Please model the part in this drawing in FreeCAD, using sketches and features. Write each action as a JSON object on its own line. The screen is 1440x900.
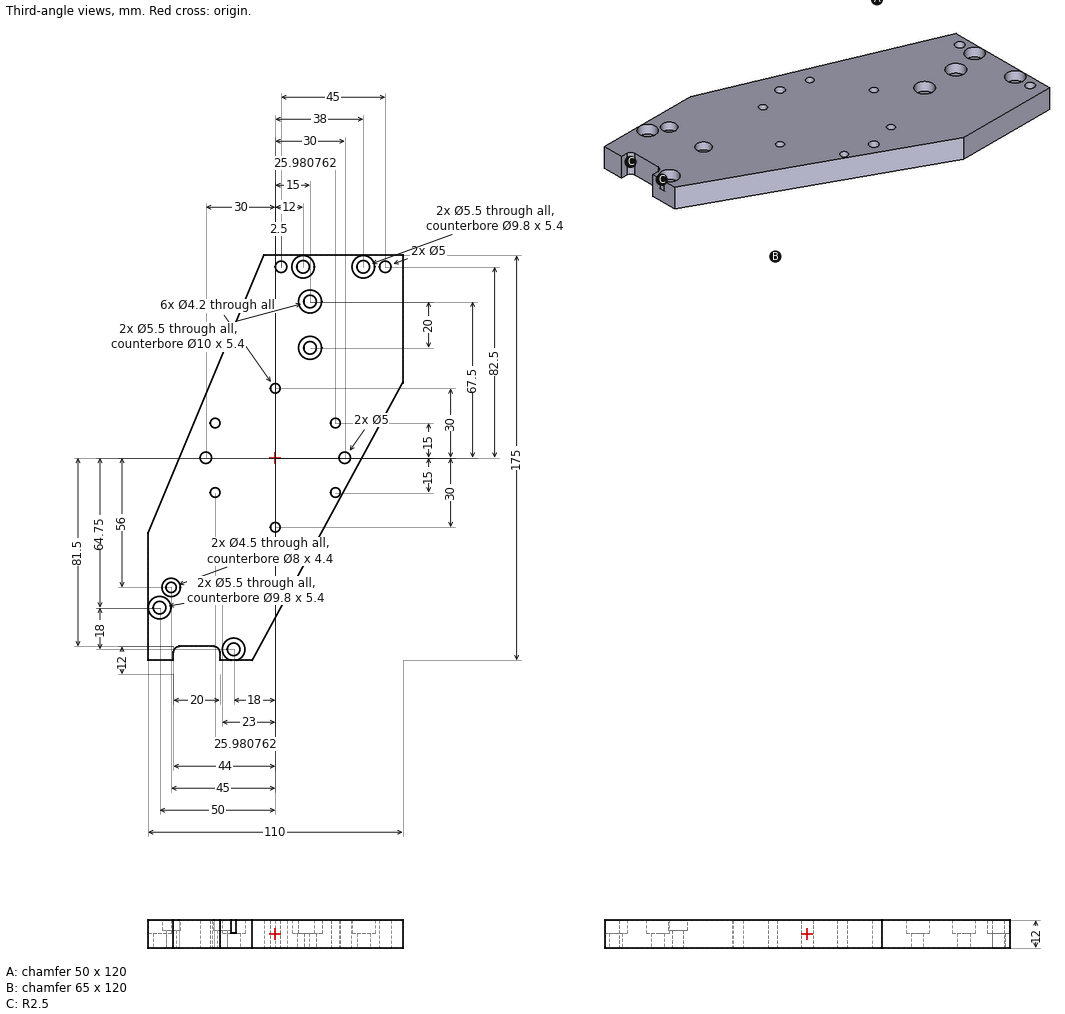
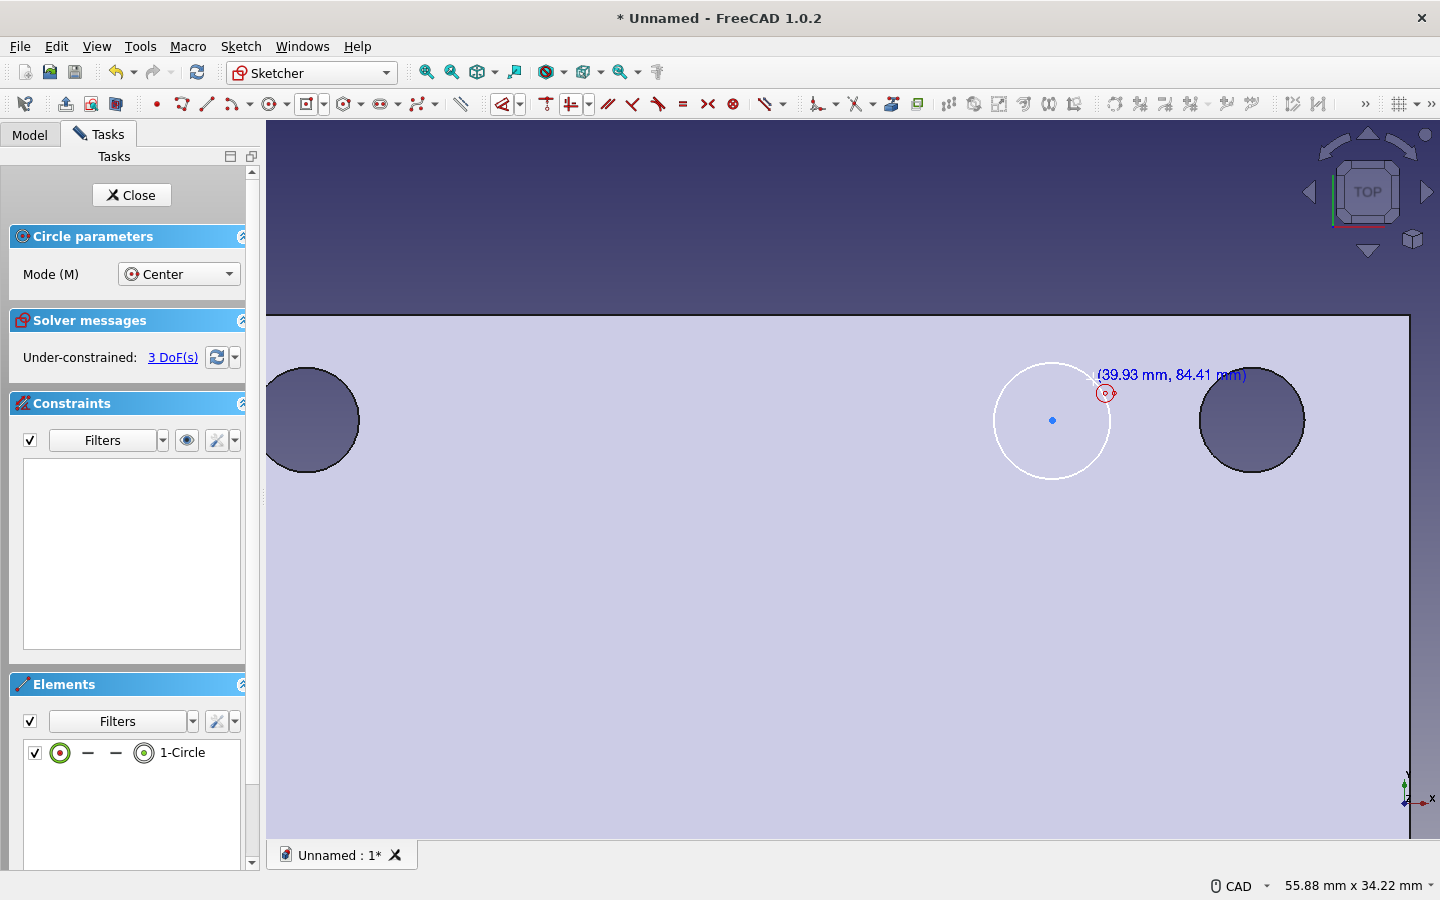
{"action": "left_click", "coordinate": [506, 420]}
{"action": "left_click", "coordinate": [547, 379]}
{"action": "key", "text": "Escape"}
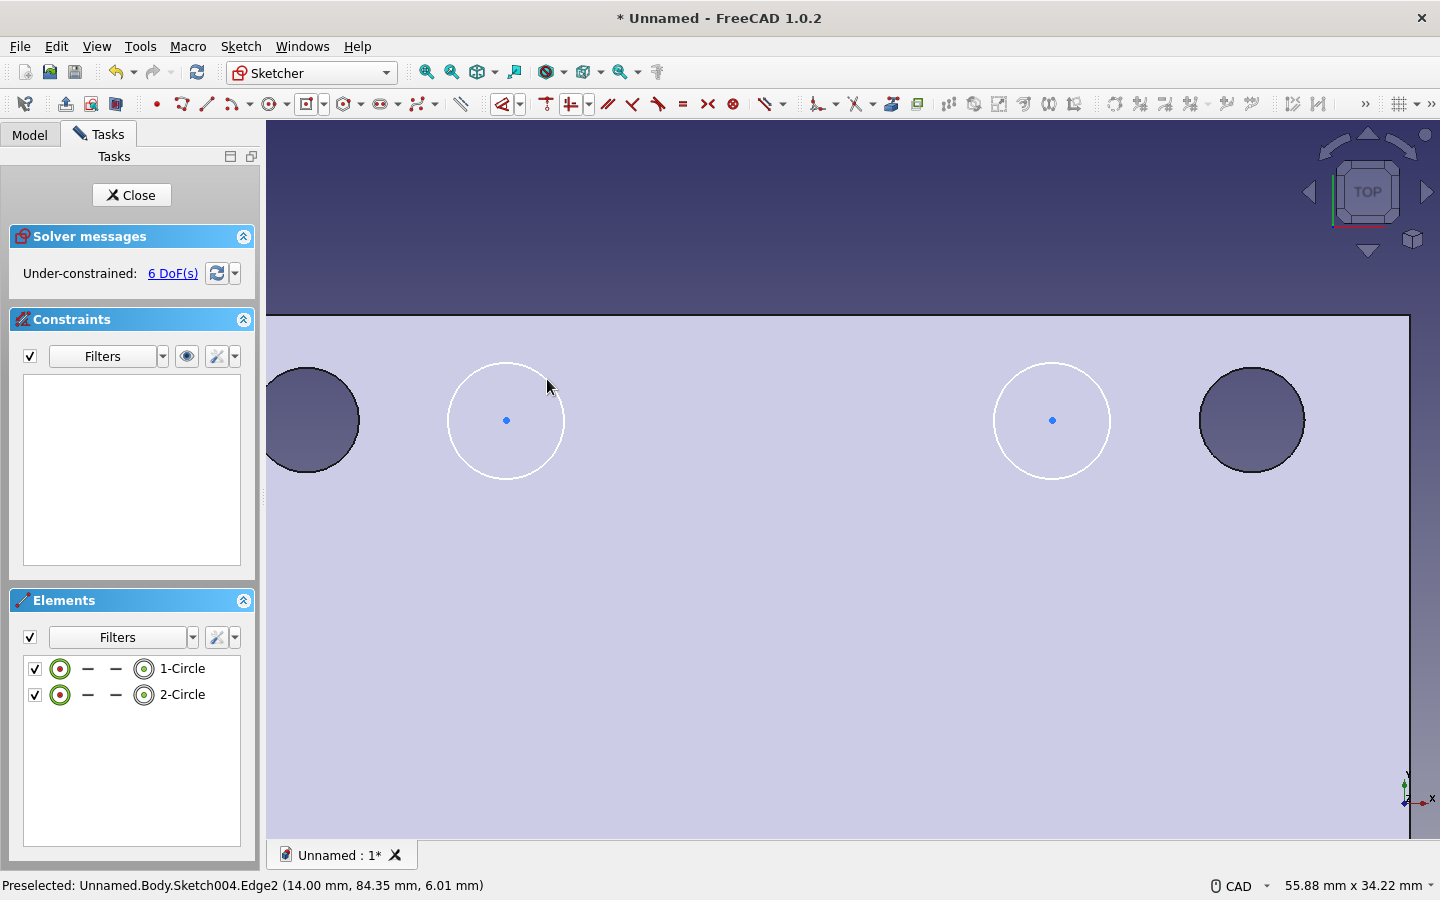
{"action": "left_click", "coordinate": [1093, 380]}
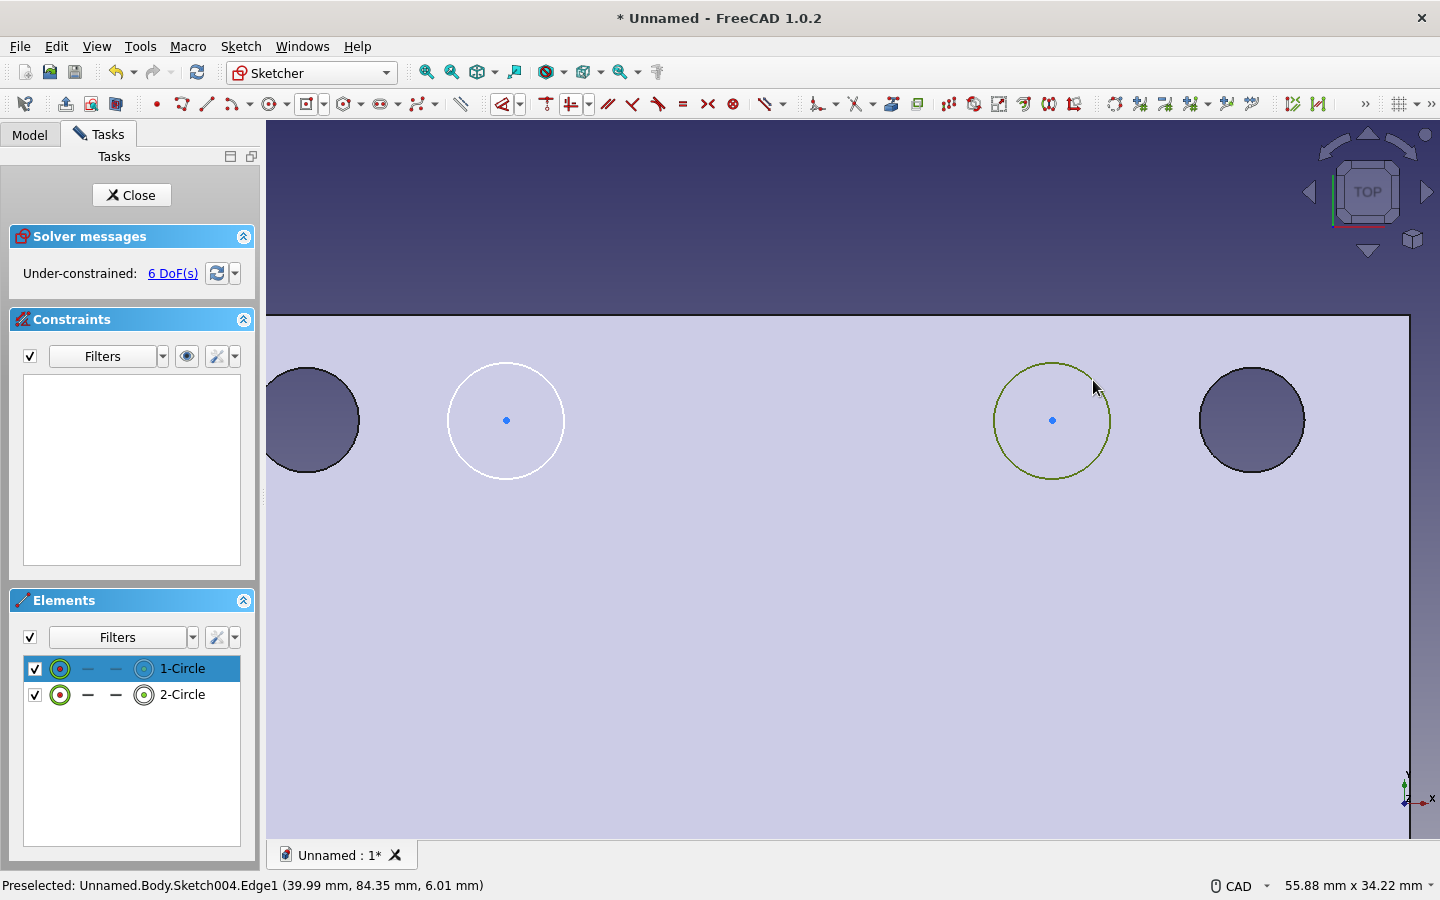
{"action": "left_click", "coordinate": [547, 380]}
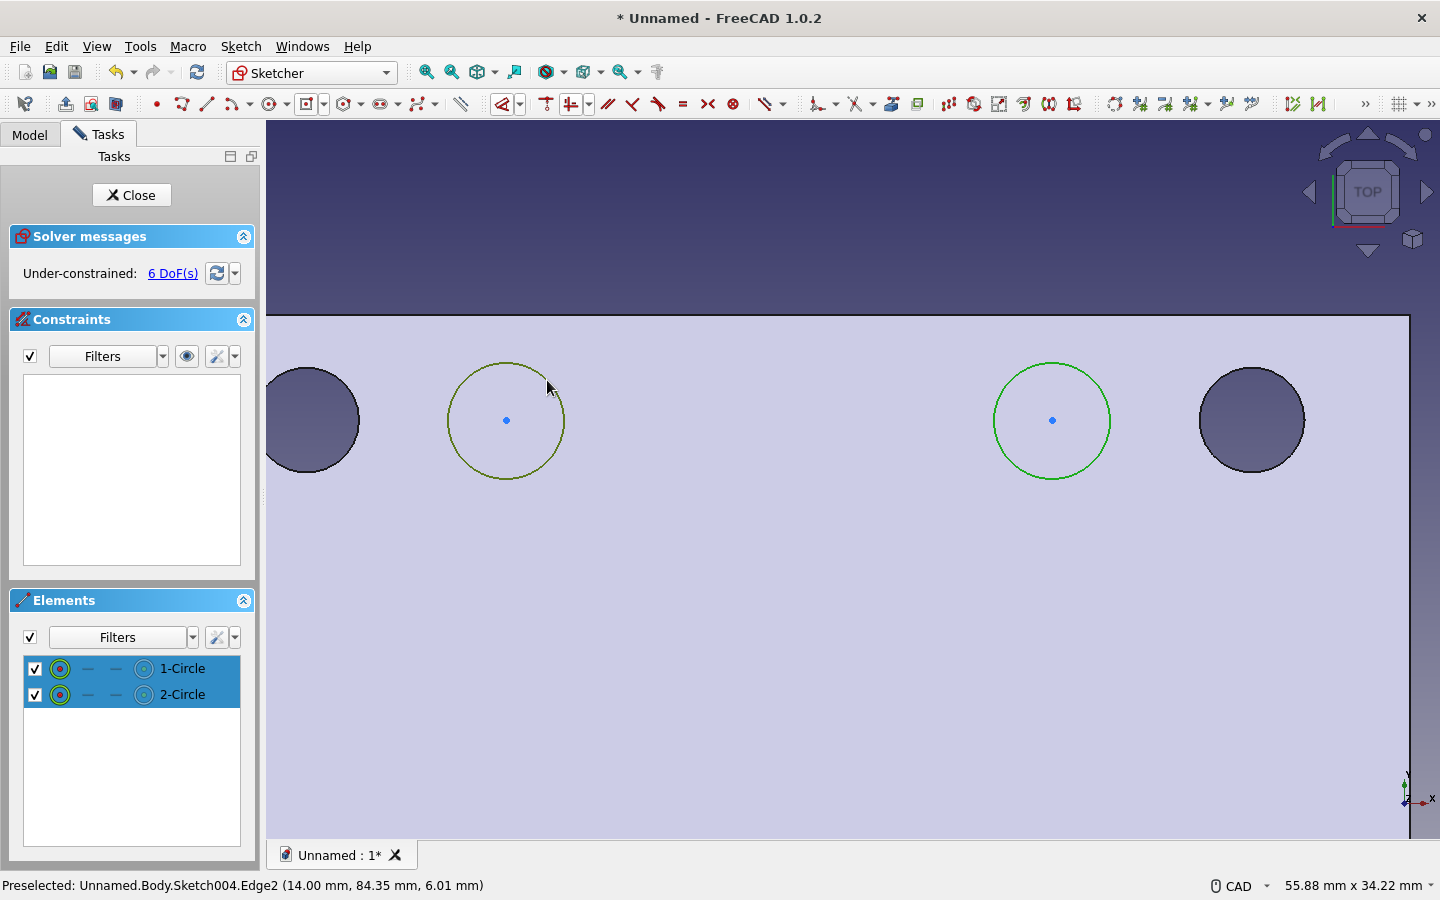
{"action": "key", "text": "e"}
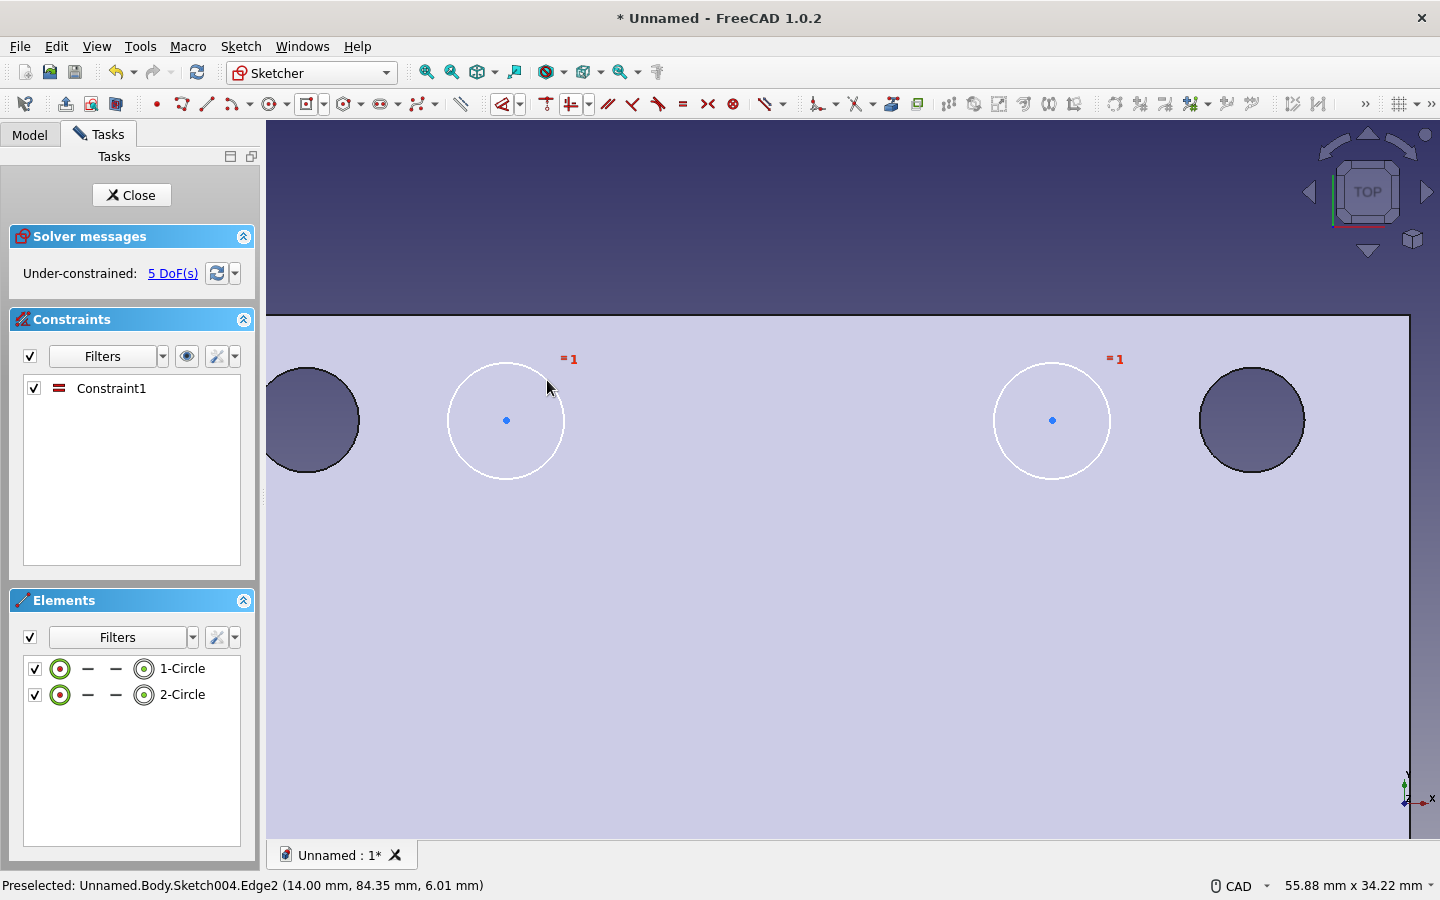
{"action": "left_click", "coordinate": [1052, 421]}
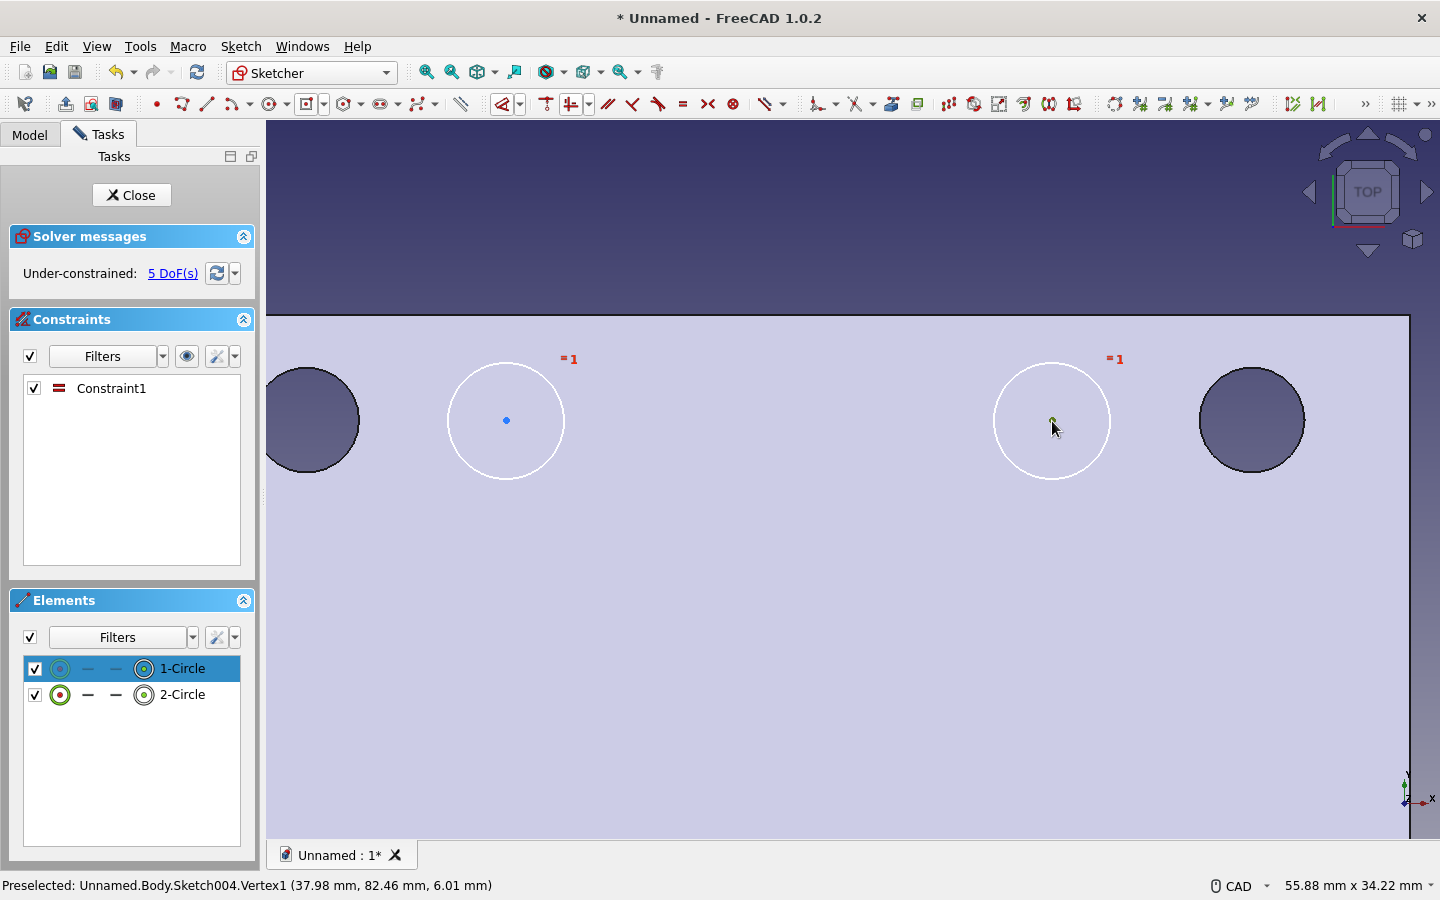
{"action": "left_click", "coordinate": [506, 421]}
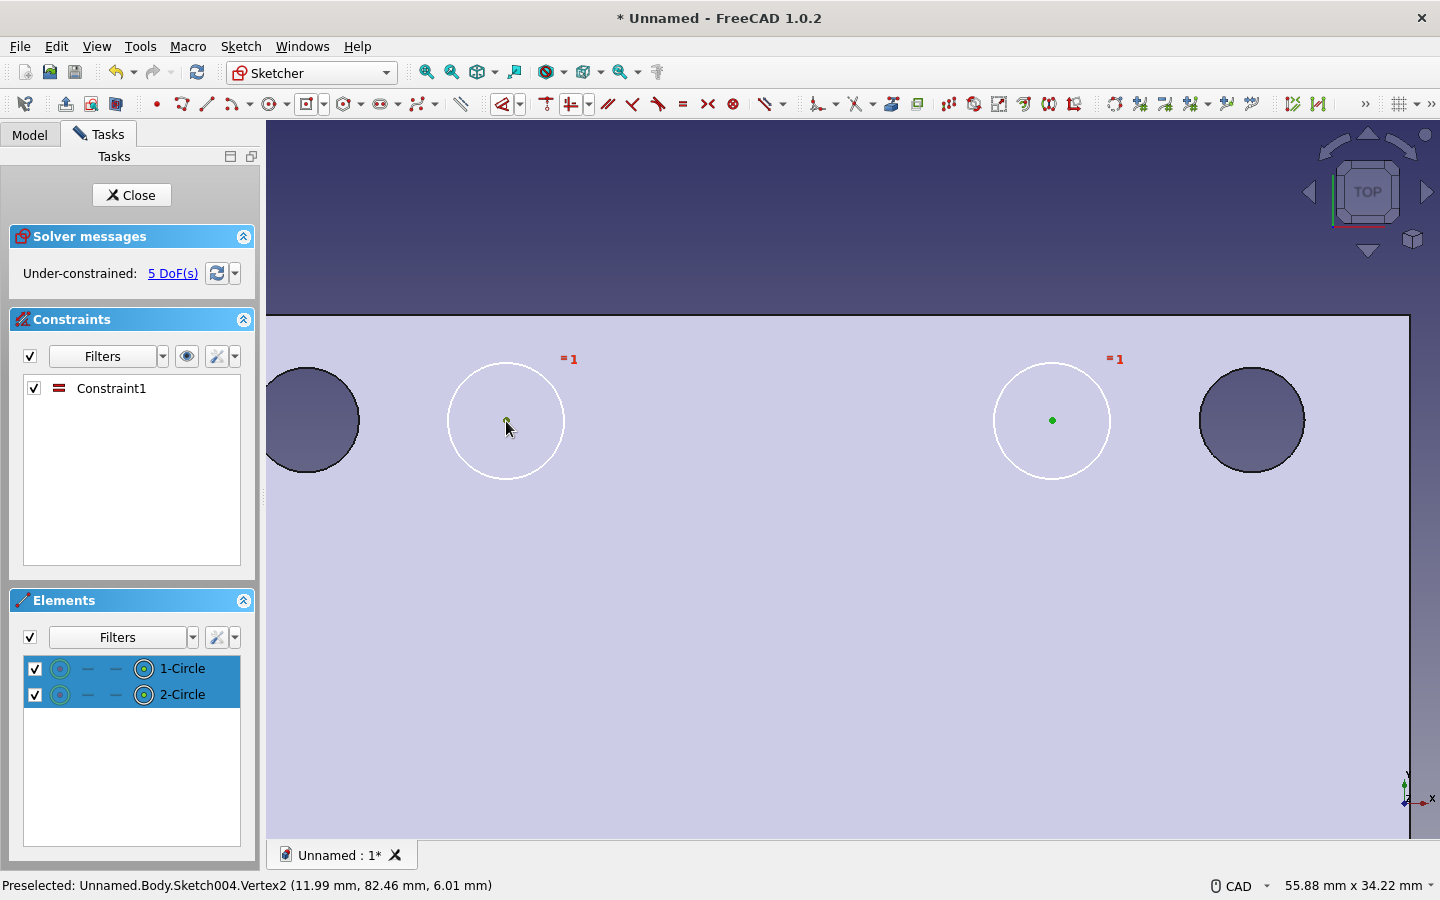
{"action": "key", "text": "h"}